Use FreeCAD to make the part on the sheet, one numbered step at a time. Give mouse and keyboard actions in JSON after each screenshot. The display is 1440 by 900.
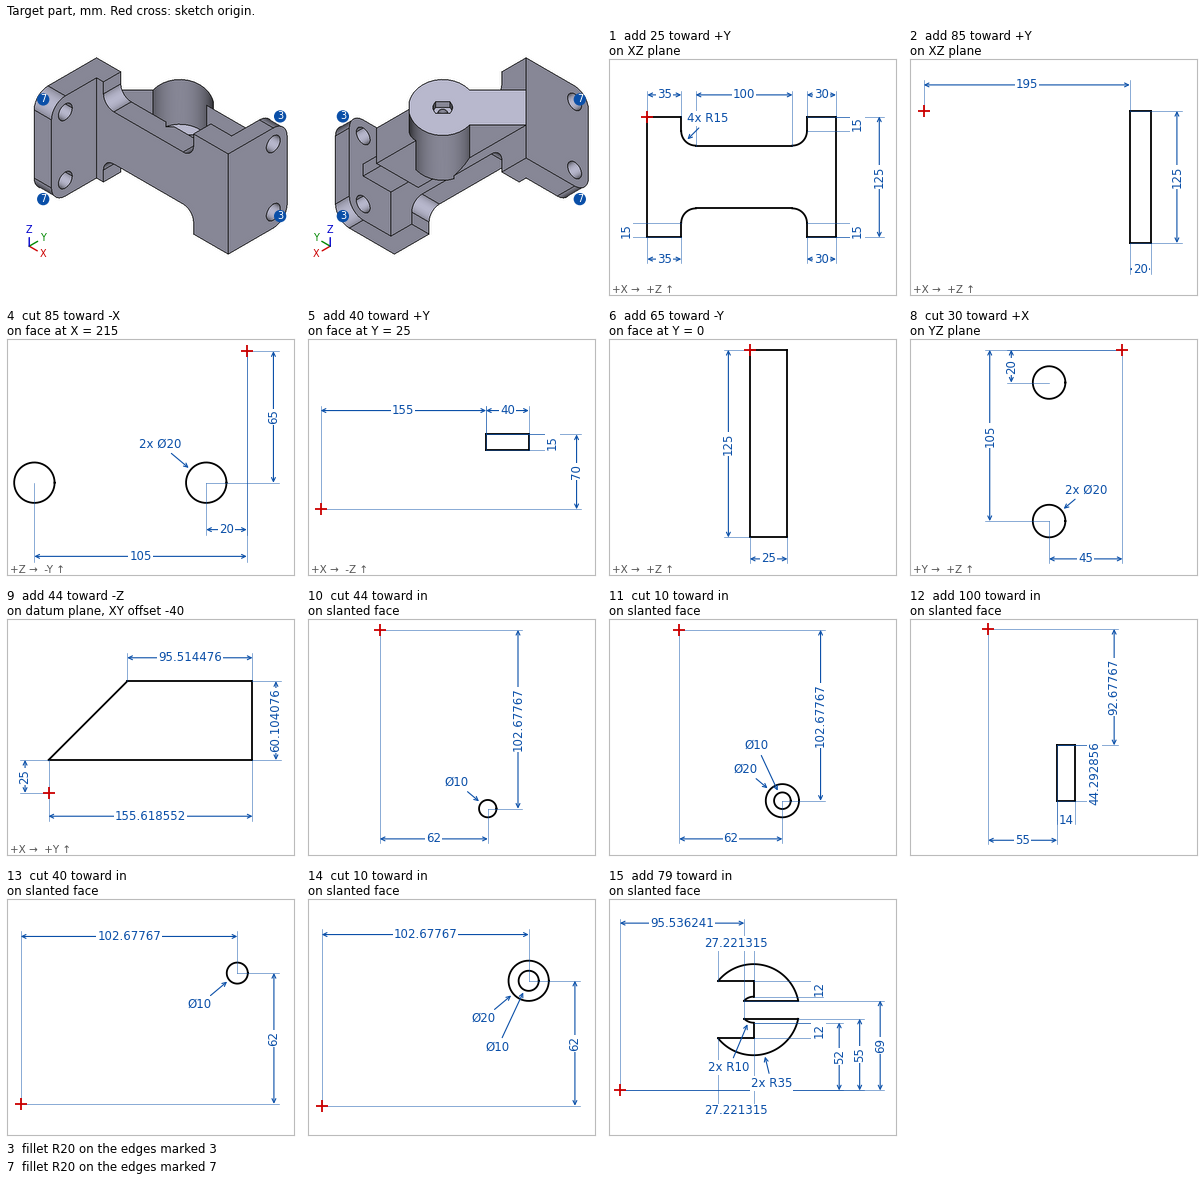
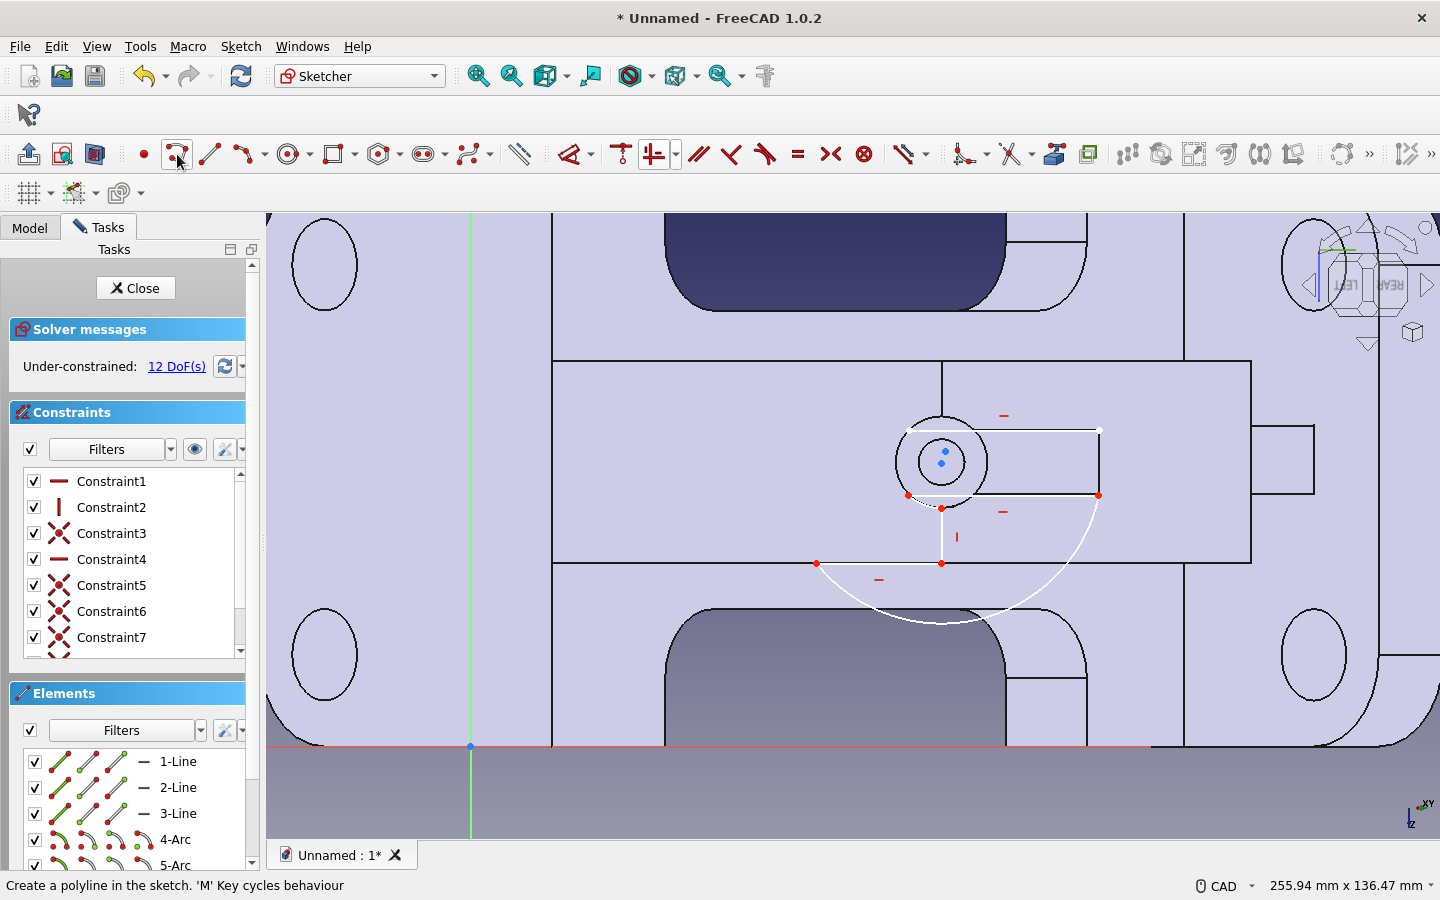
{"action": "left_click", "coordinate": [817, 361]}
{"action": "left_click", "coordinate": [942, 361]}
{"action": "left_click", "coordinate": [942, 416]}
{"action": "right_click", "coordinate": [942, 416]}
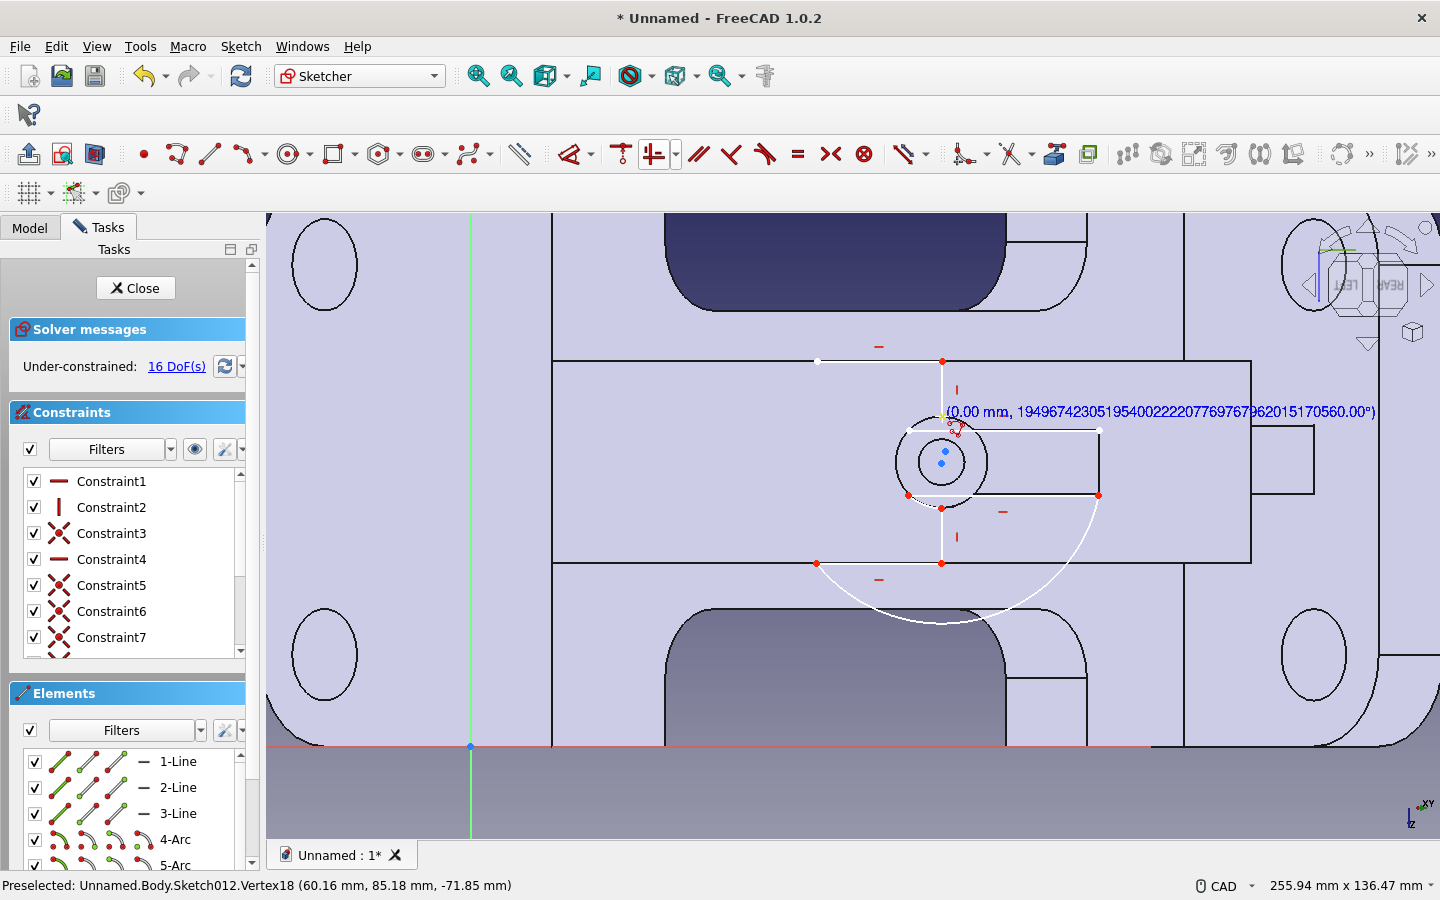
{"action": "left_click", "coordinate": [242, 154]}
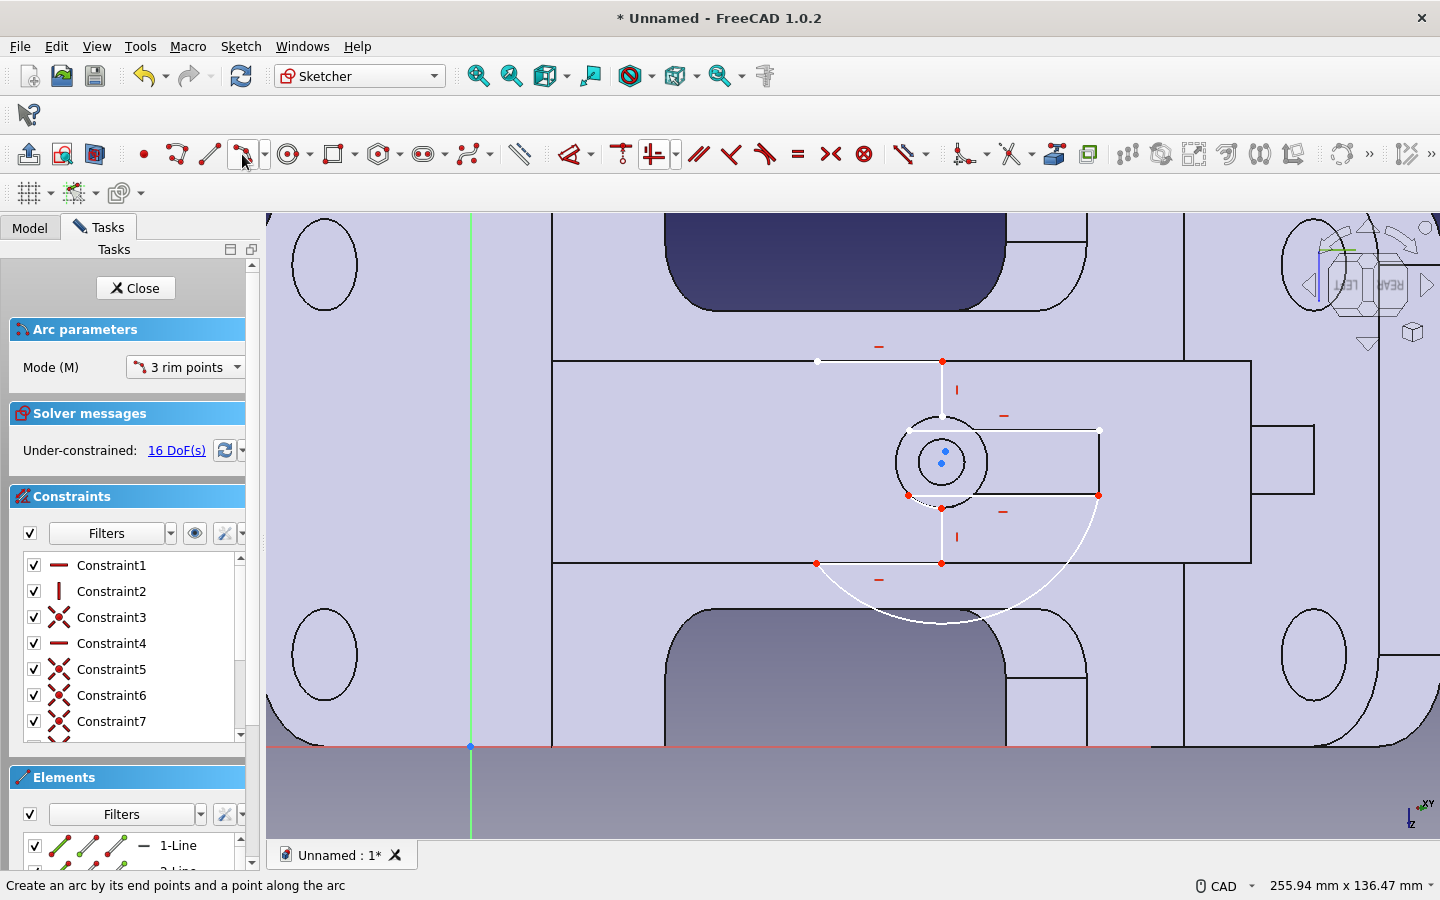
{"action": "left_click", "coordinate": [1099, 431]}
{"action": "left_click", "coordinate": [817, 362]}
{"action": "left_click", "coordinate": [980, 306]}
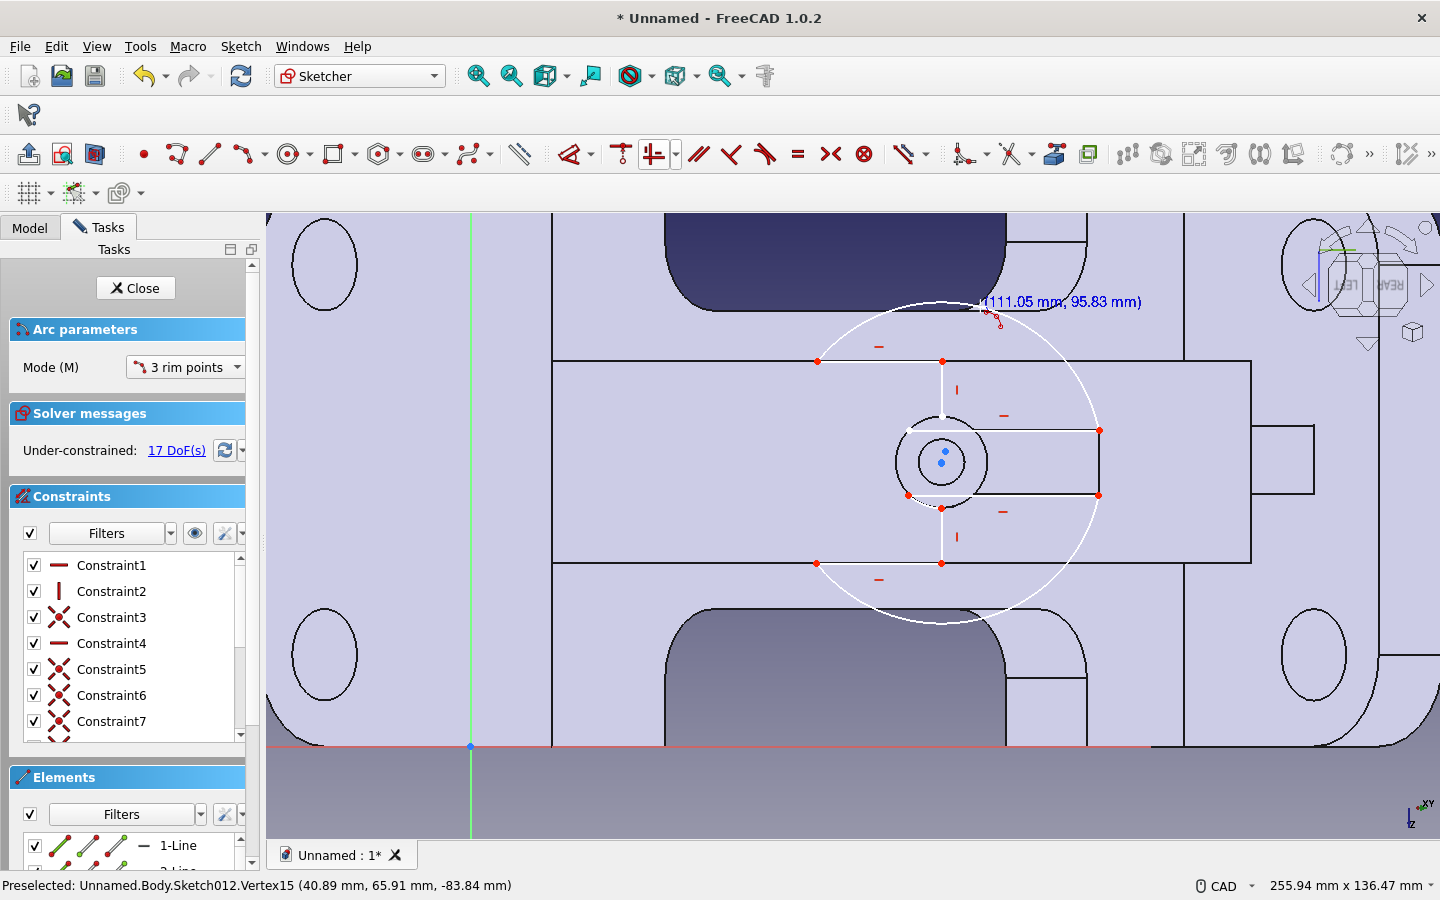
{"action": "left_click", "coordinate": [942, 417]}
{"action": "left_click", "coordinate": [909, 431]}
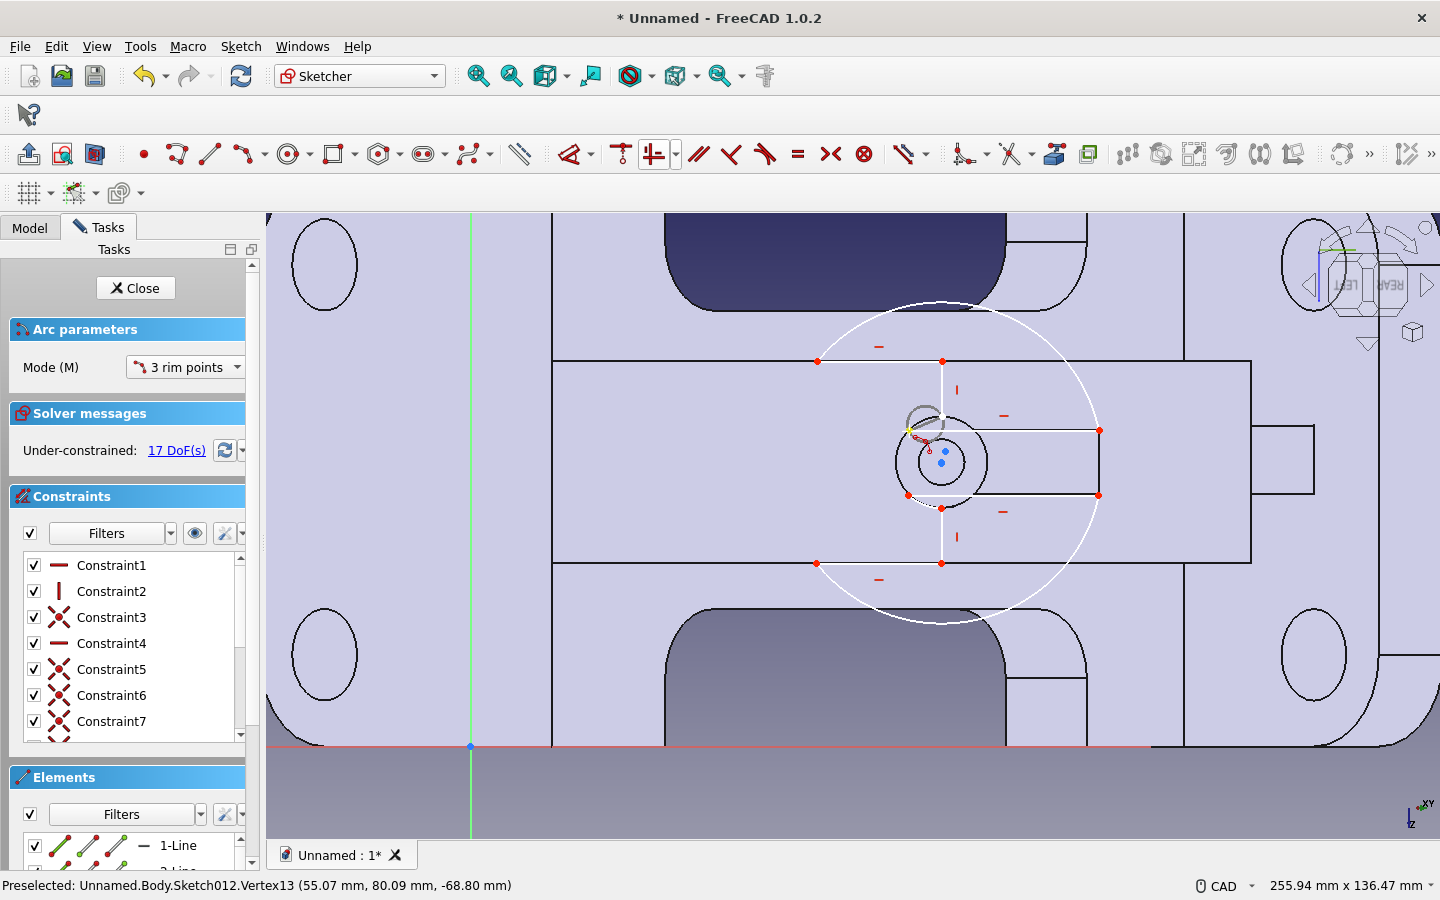
{"action": "scroll", "coordinate": [924, 420], "scroll_direction": "up", "scroll_amount": 8}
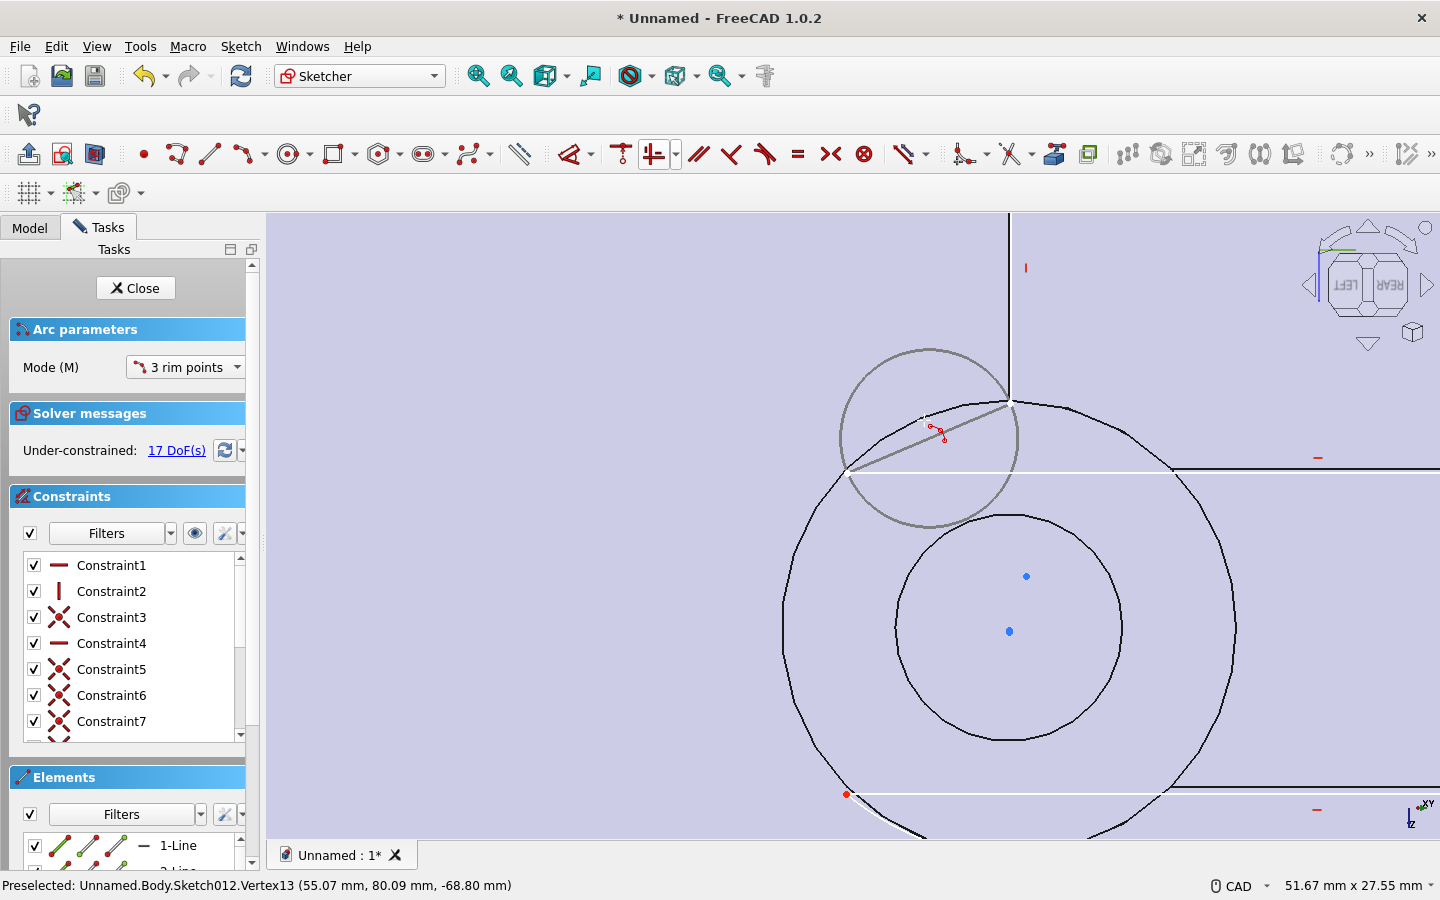
{"action": "left_click", "coordinate": [921, 418]}
{"action": "key", "text": "Escape"}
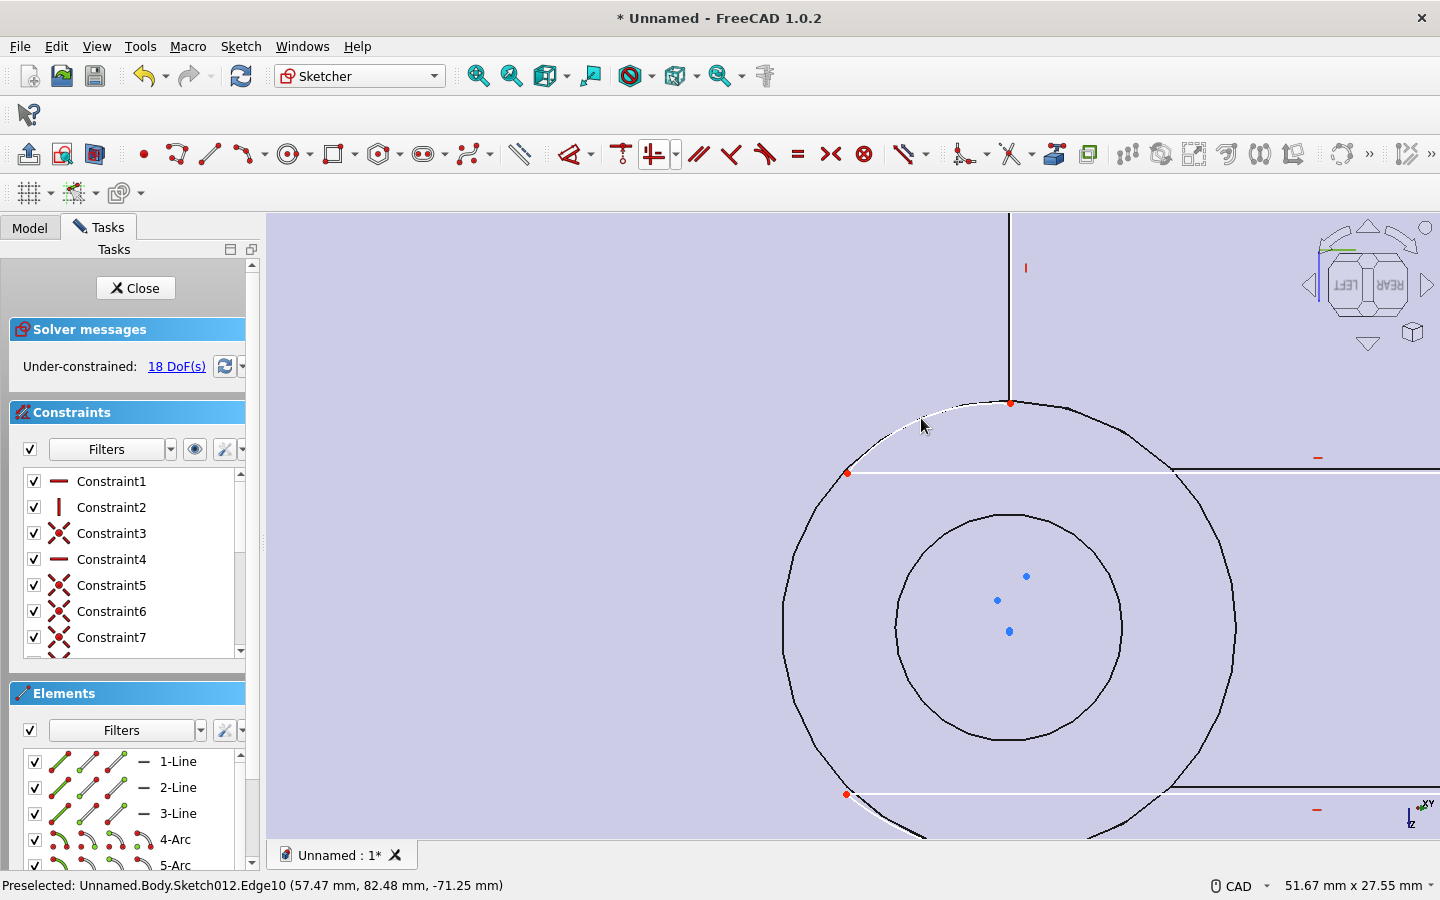
{"action": "scroll", "coordinate": [924, 420], "scroll_direction": "down", "scroll_amount": 8}